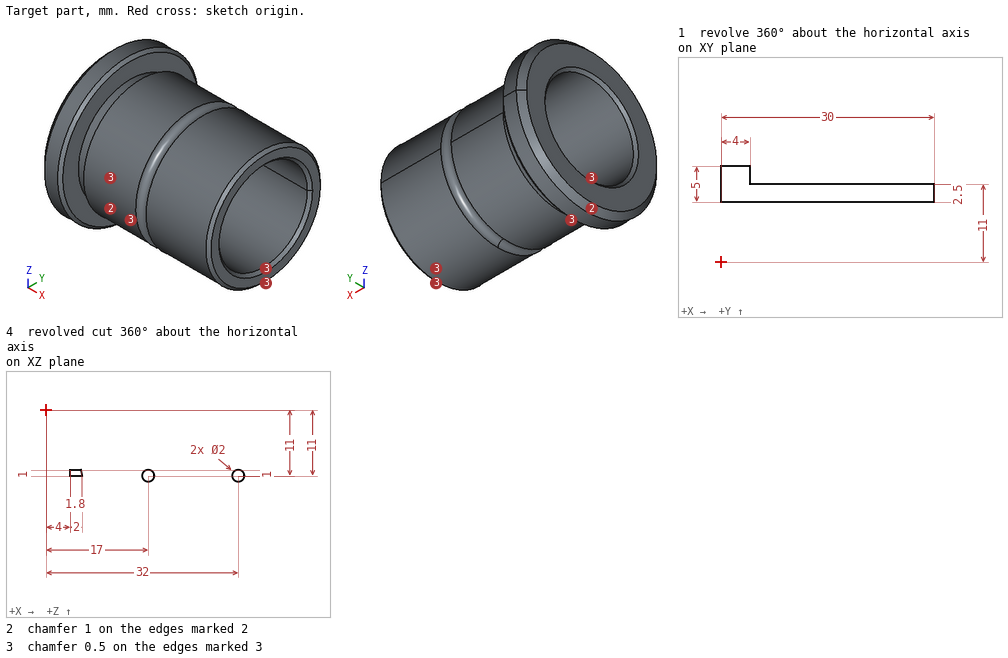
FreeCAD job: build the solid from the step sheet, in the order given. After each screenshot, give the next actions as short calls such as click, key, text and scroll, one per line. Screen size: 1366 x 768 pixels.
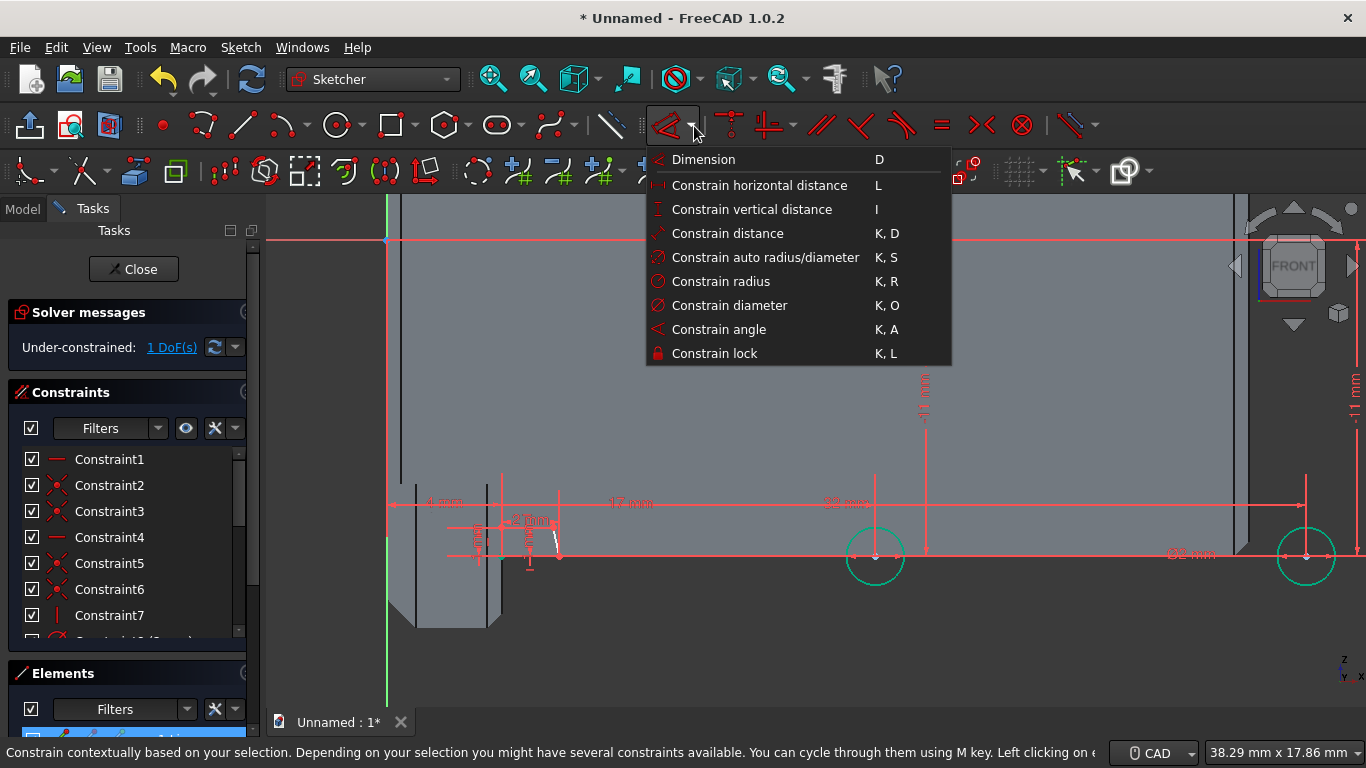
click(799, 185)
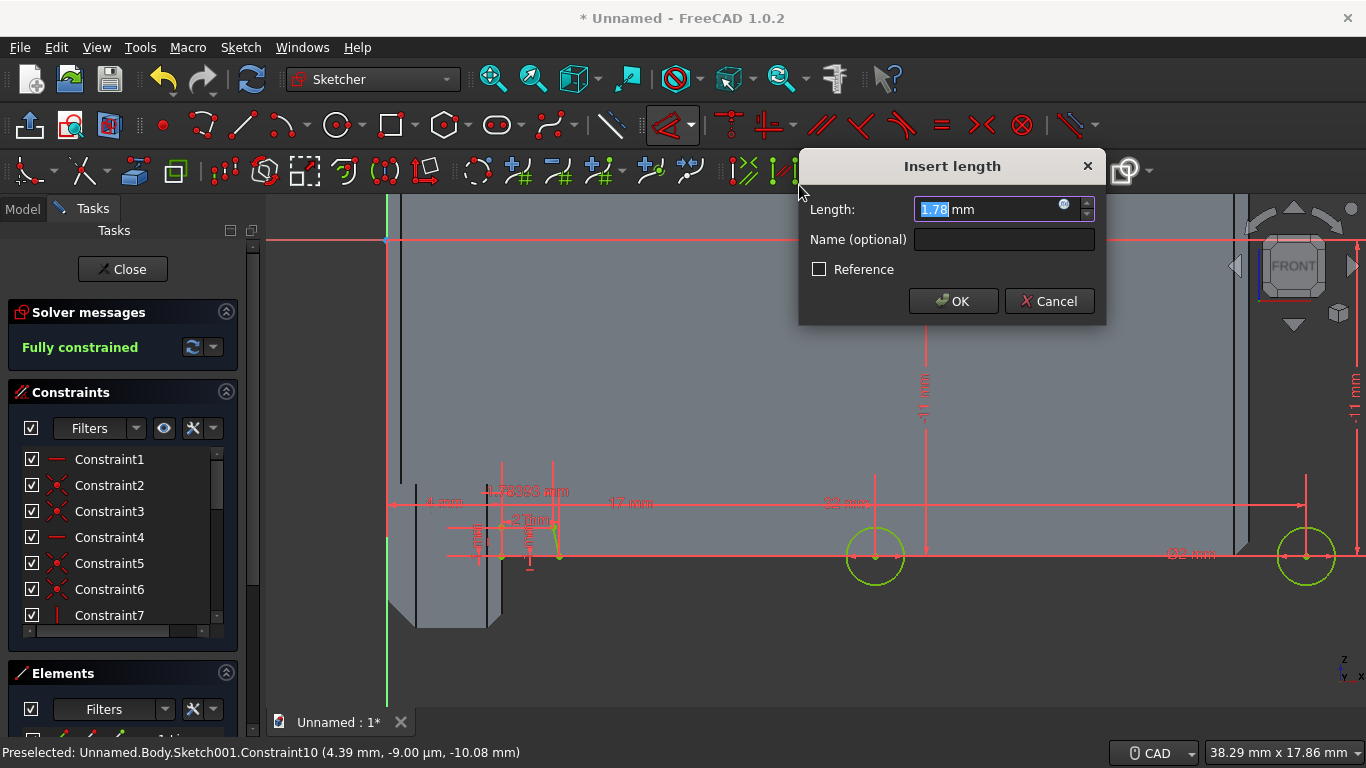
text(1.8)
key(Return)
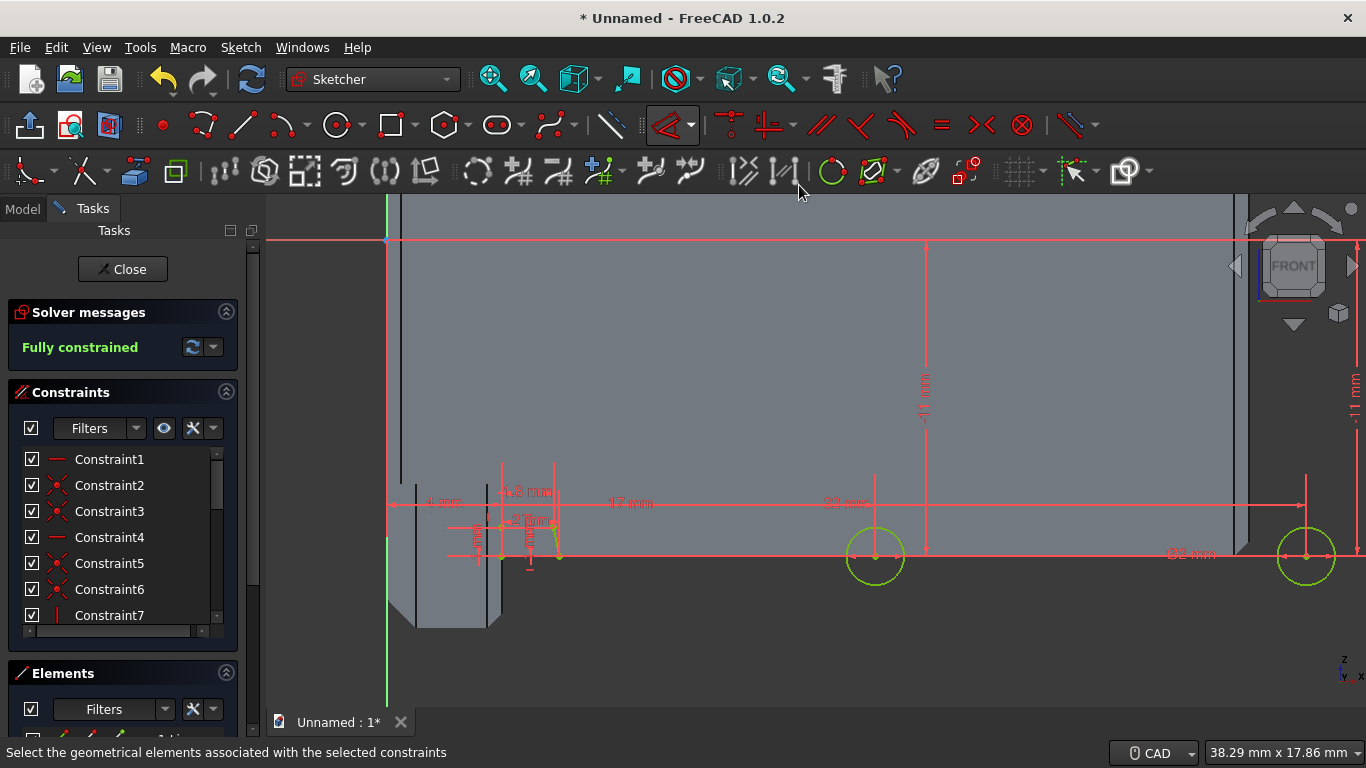
click(123, 269)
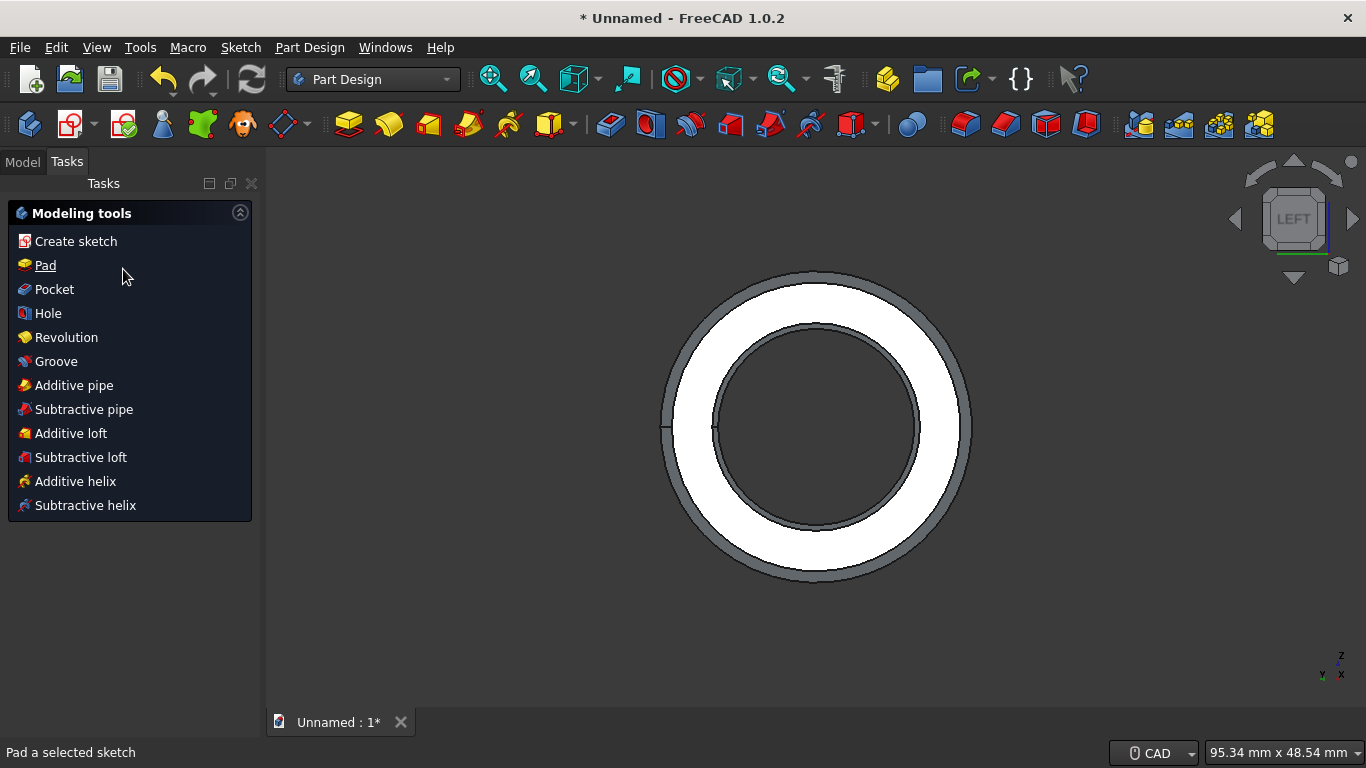
click(692, 124)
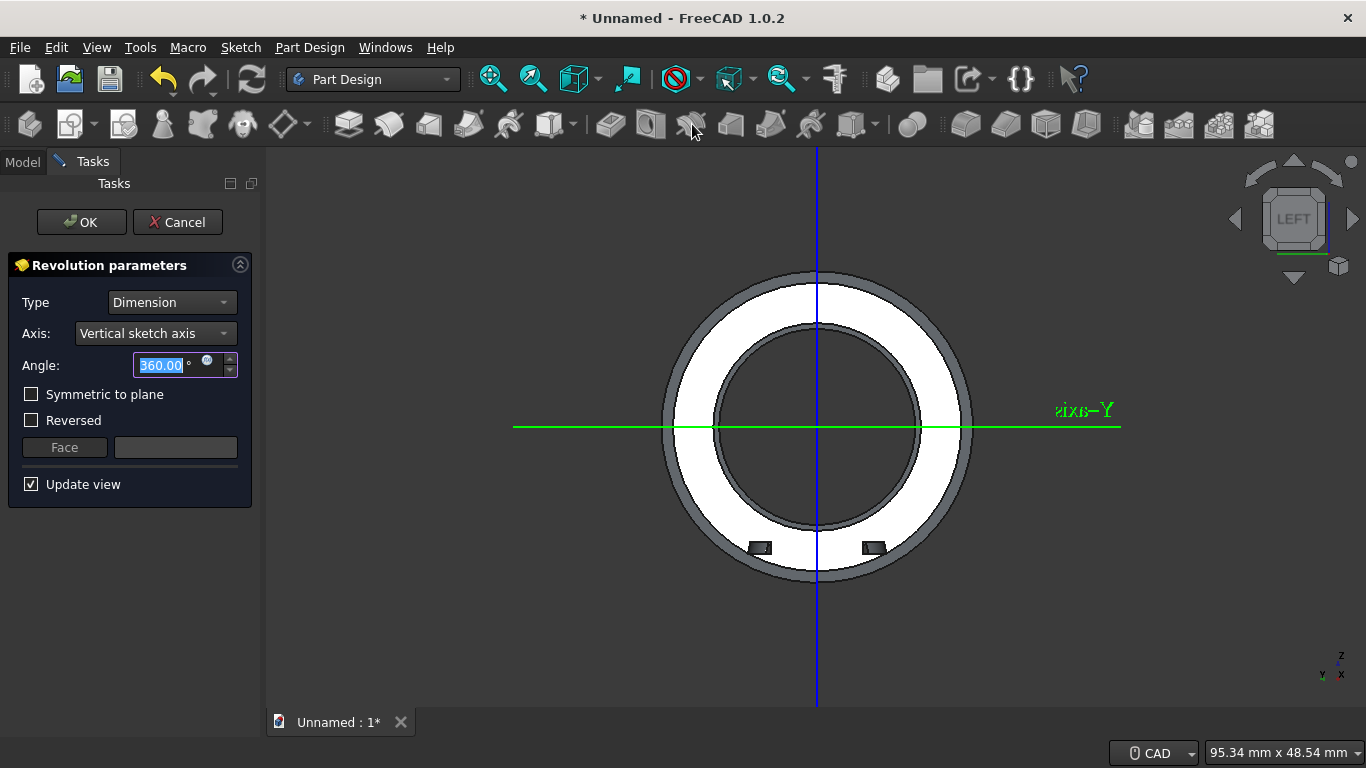
click(156, 334)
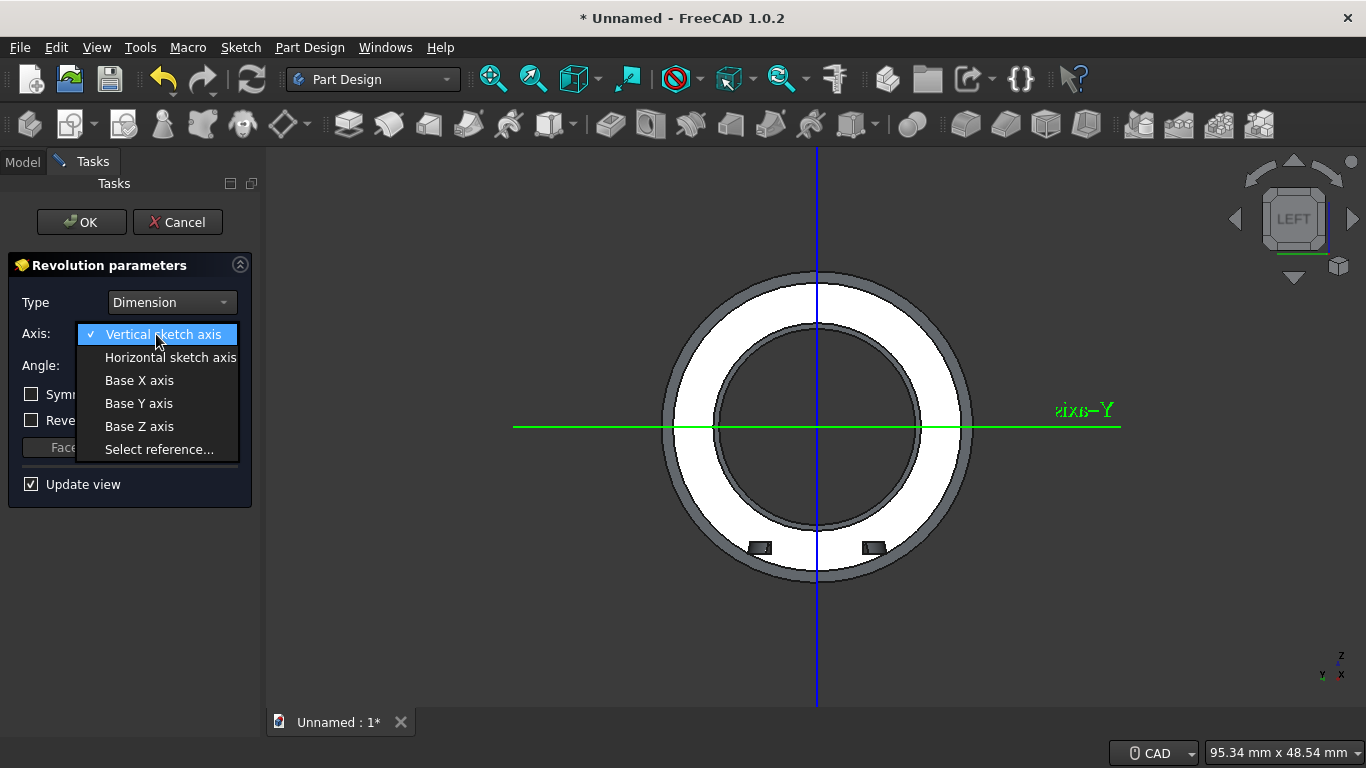
click(156, 358)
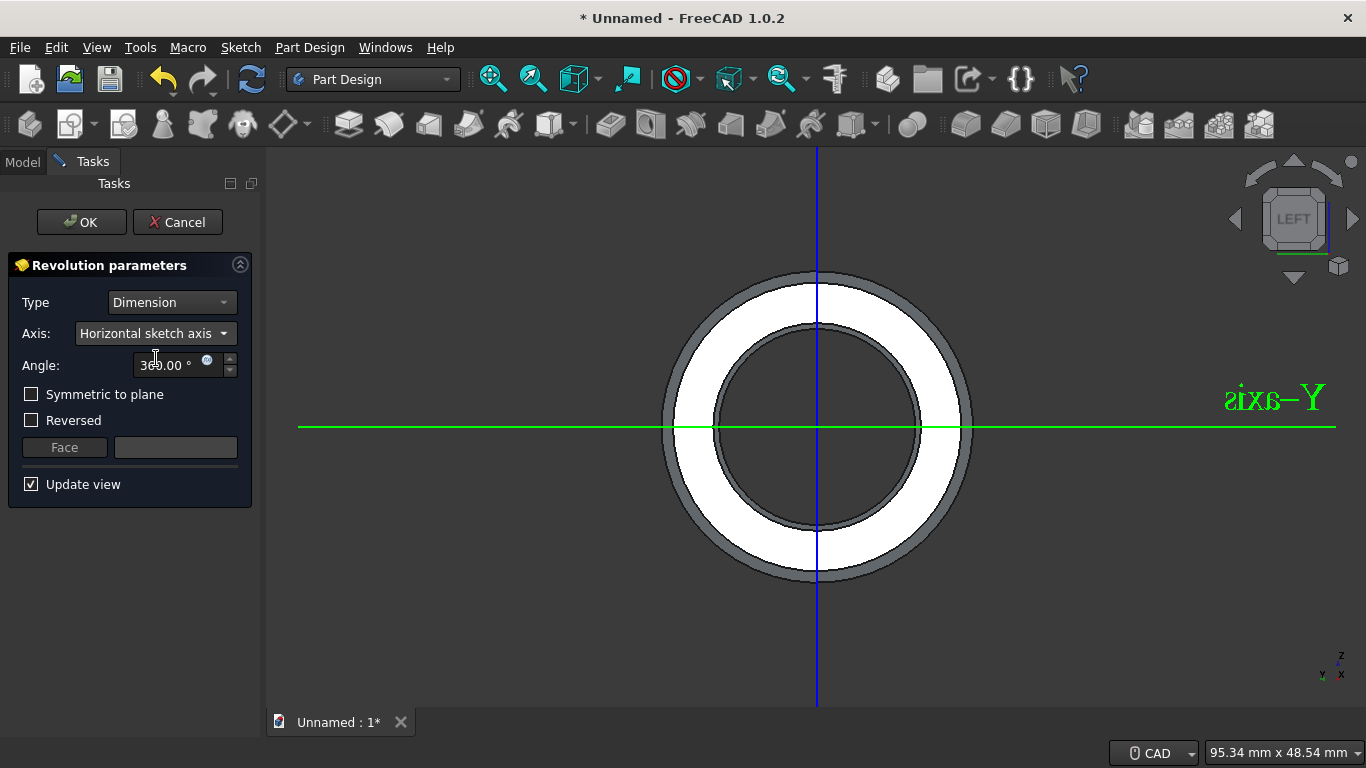
click(82, 222)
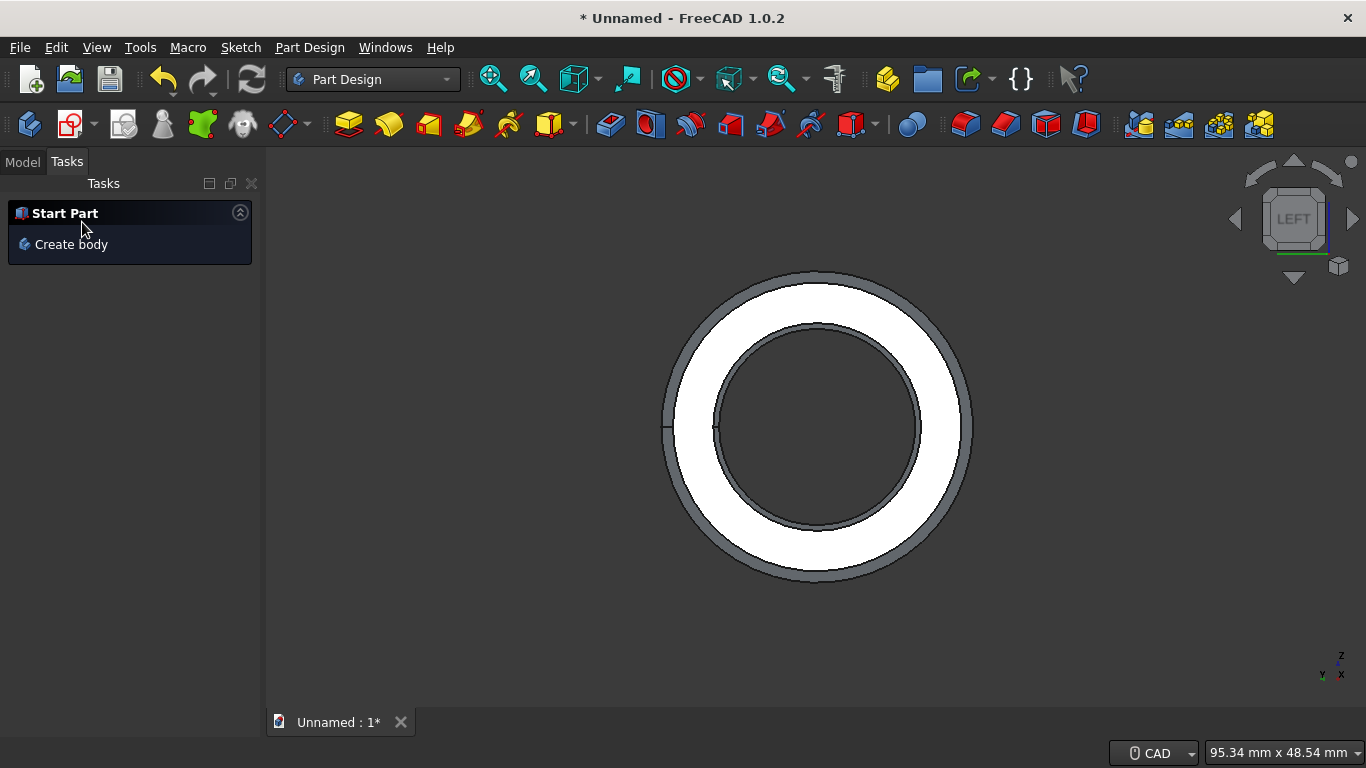
key(0)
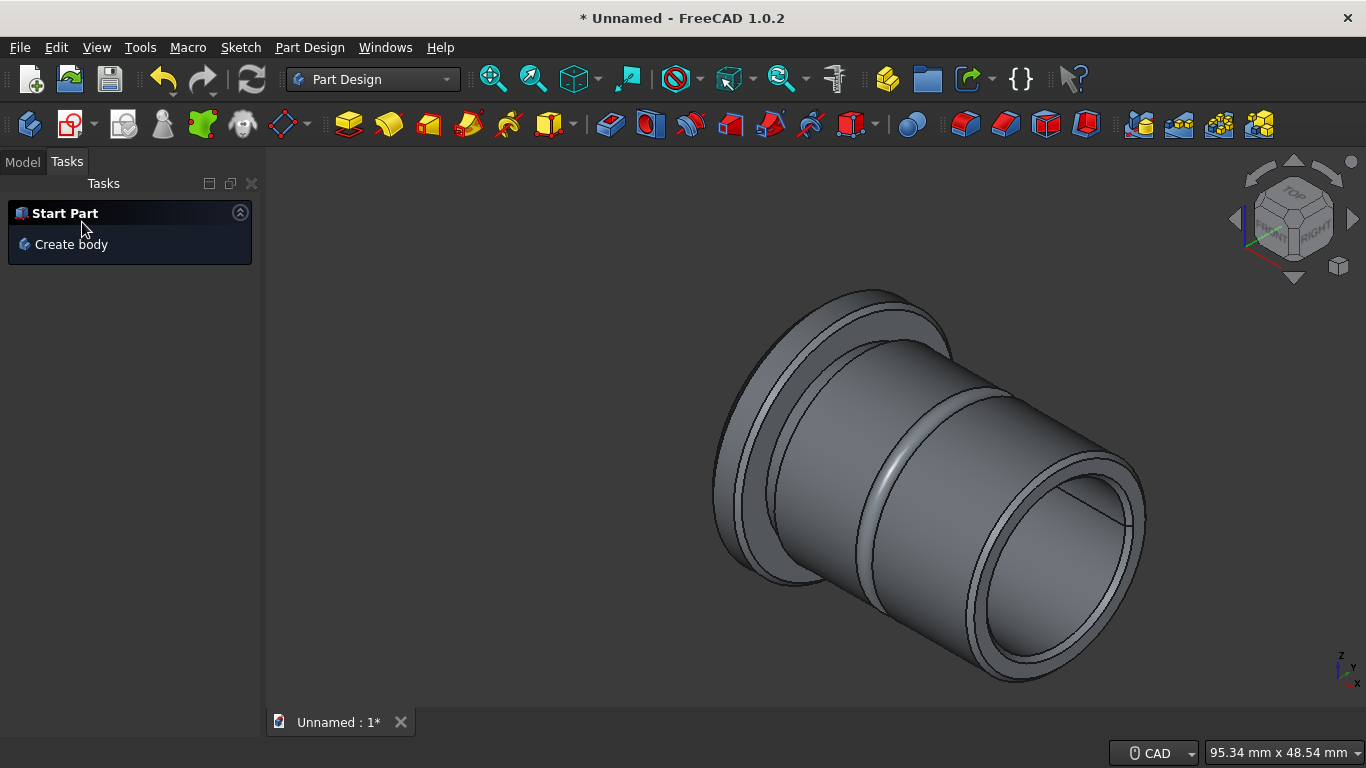
click(494, 80)